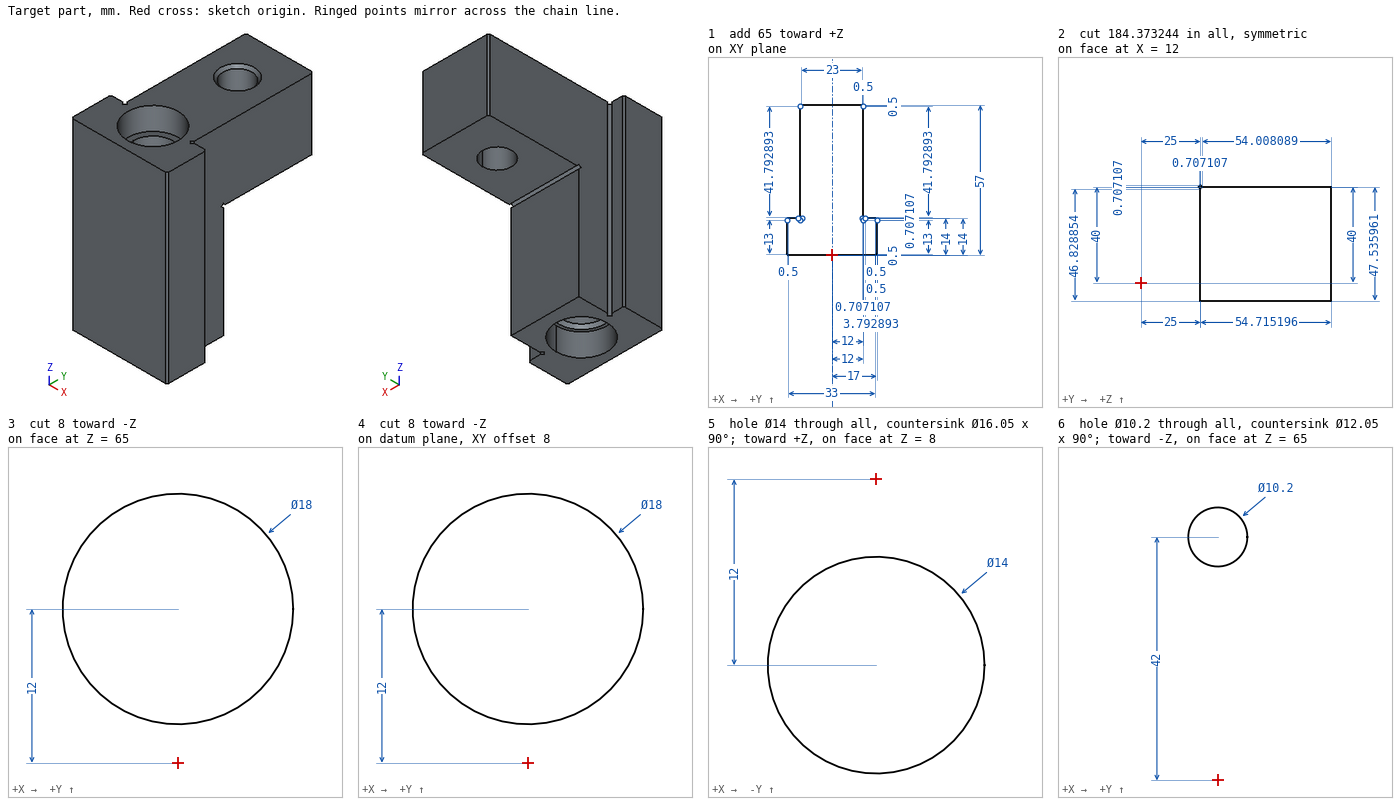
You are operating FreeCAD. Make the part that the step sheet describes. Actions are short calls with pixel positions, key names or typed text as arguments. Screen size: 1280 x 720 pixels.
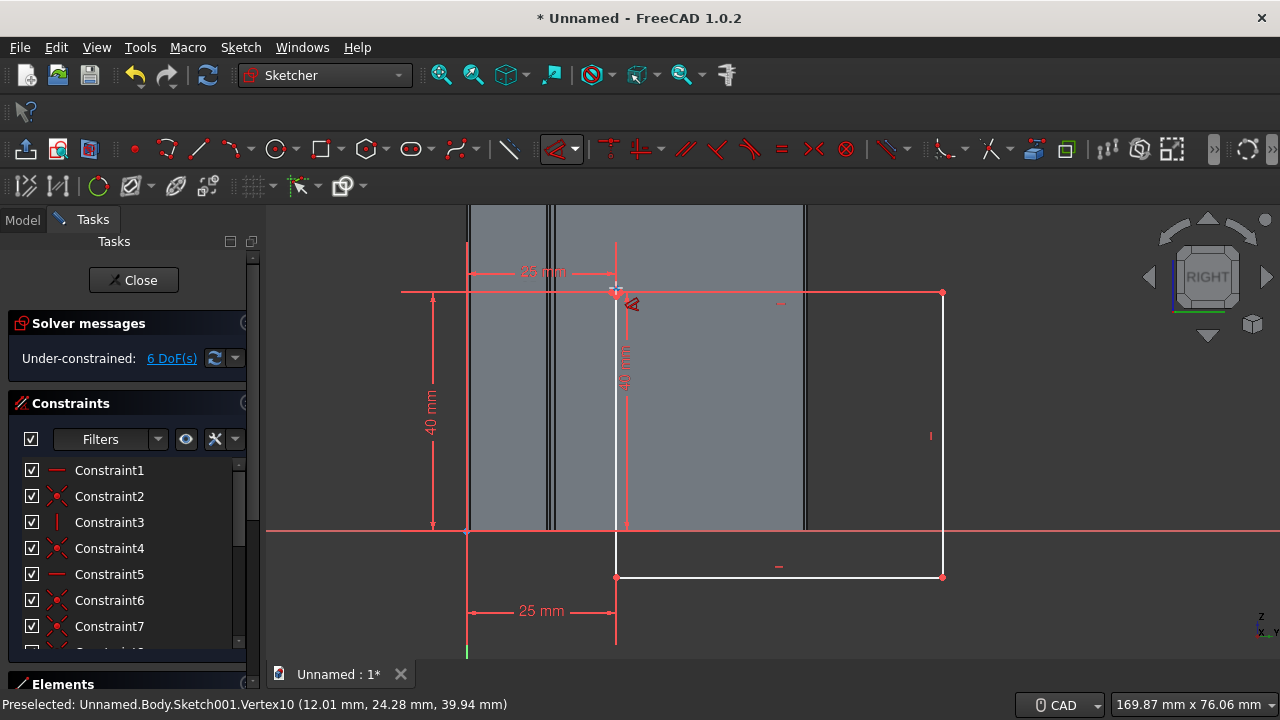
click(714, 578)
click(779, 612)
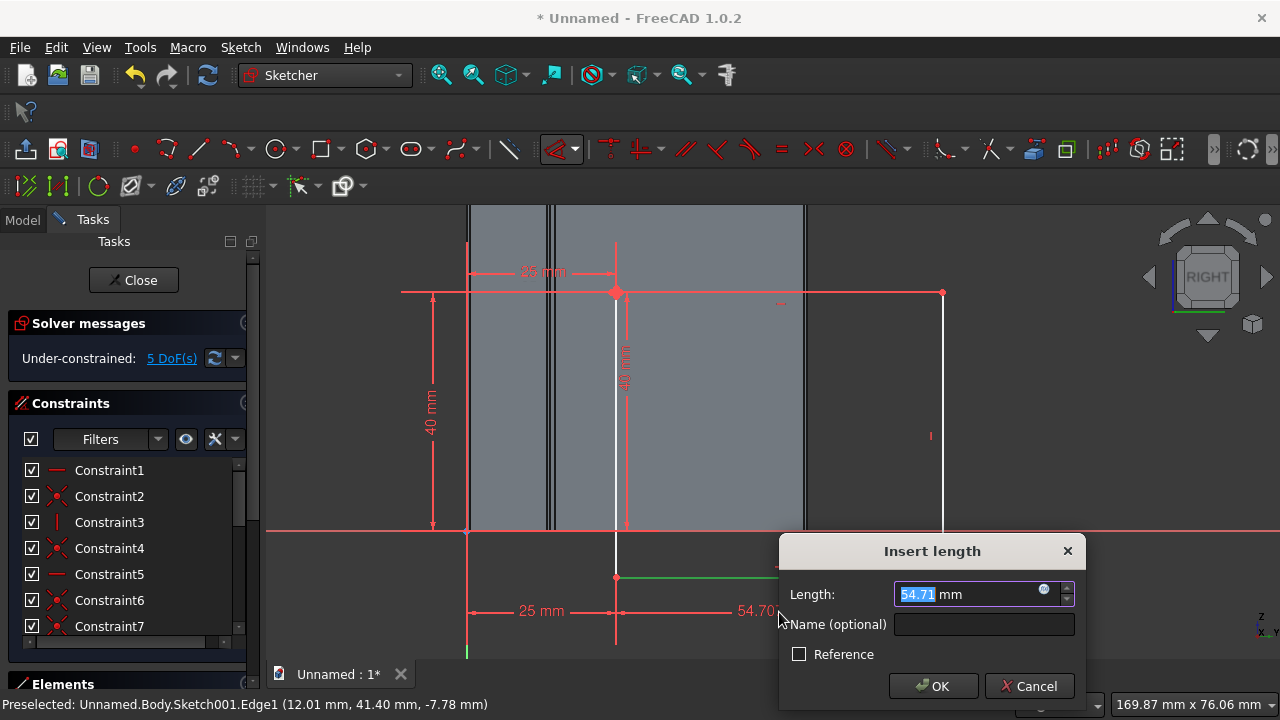
text(54.715196)
key(Return)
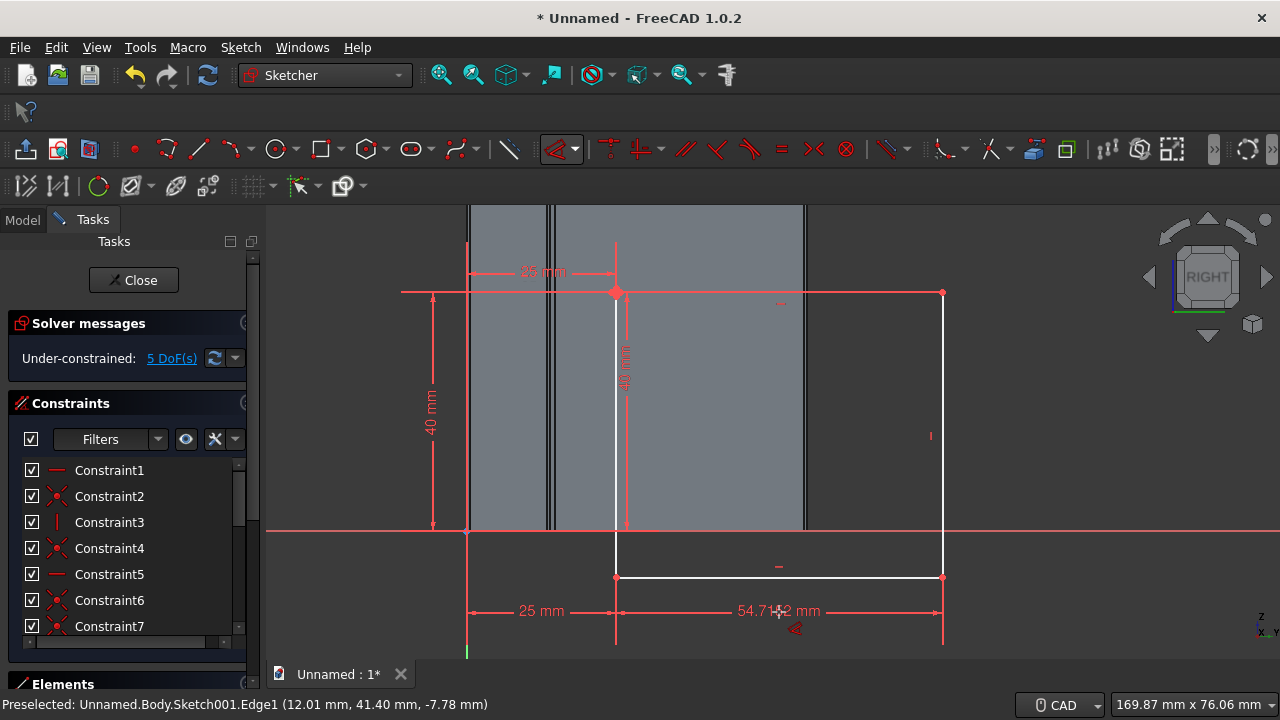
click(943, 492)
click(977, 435)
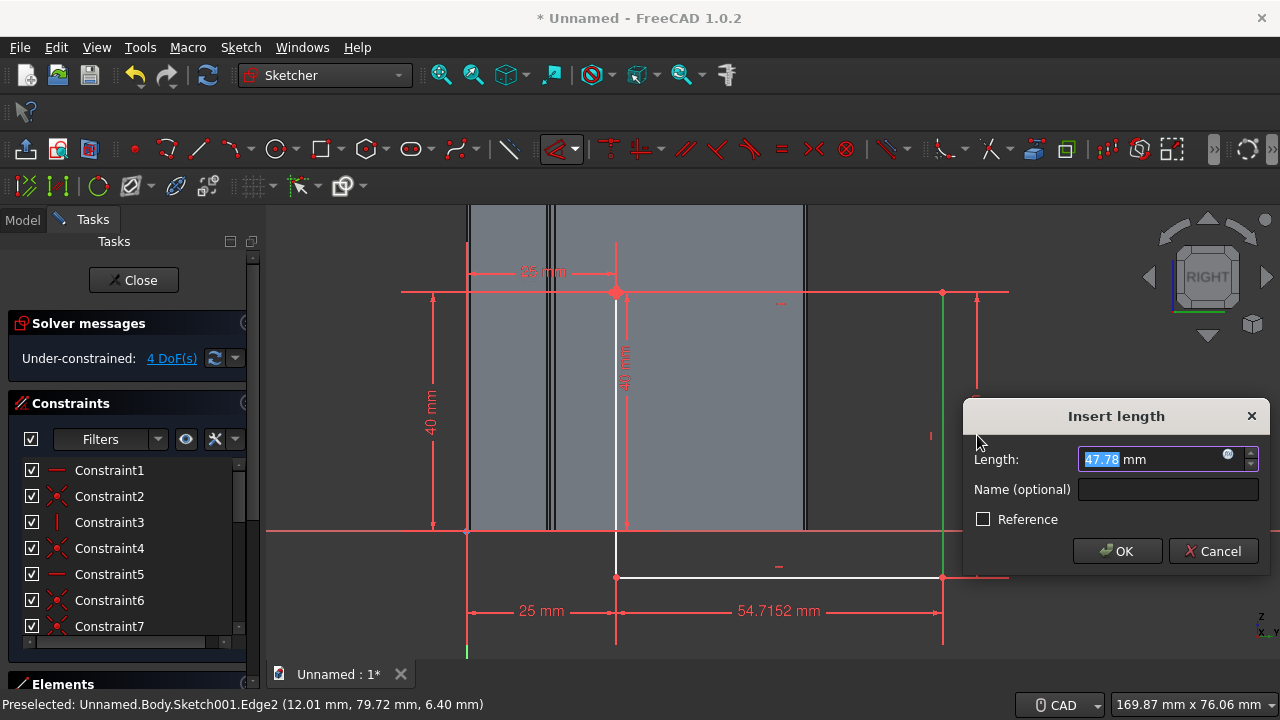
text(47.535961)
key(Return)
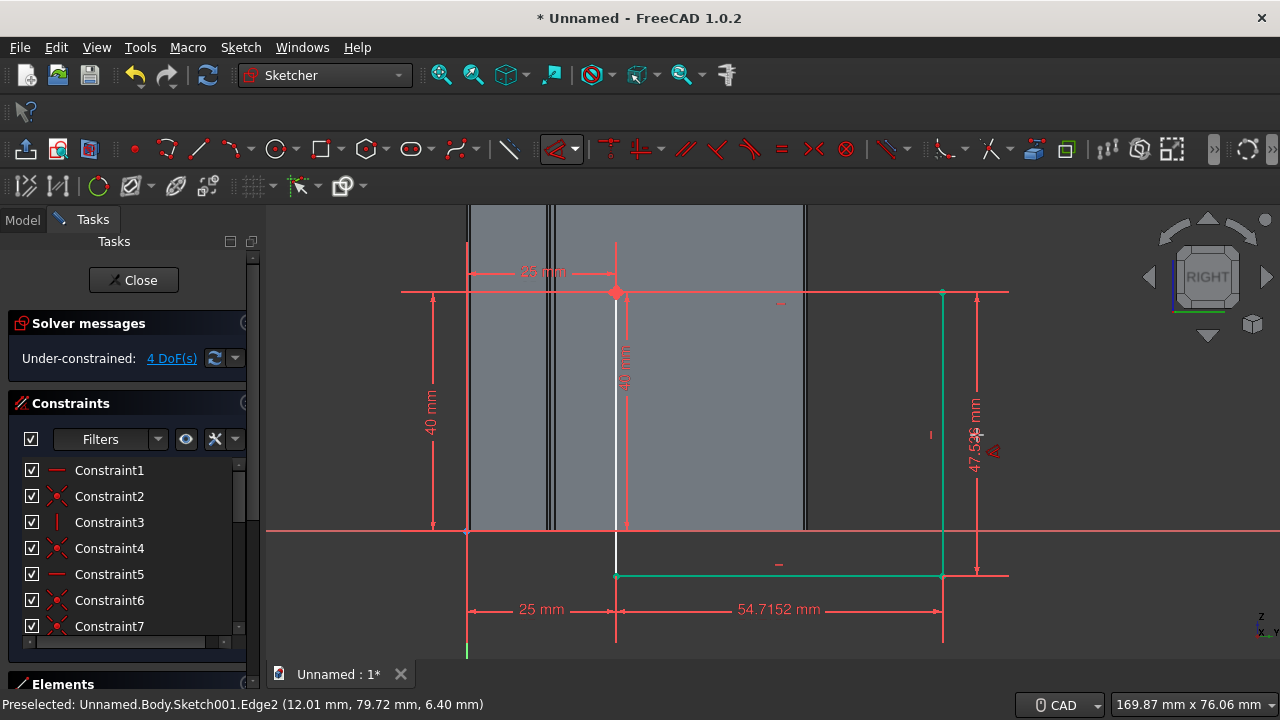
click(846, 292)
click(782, 258)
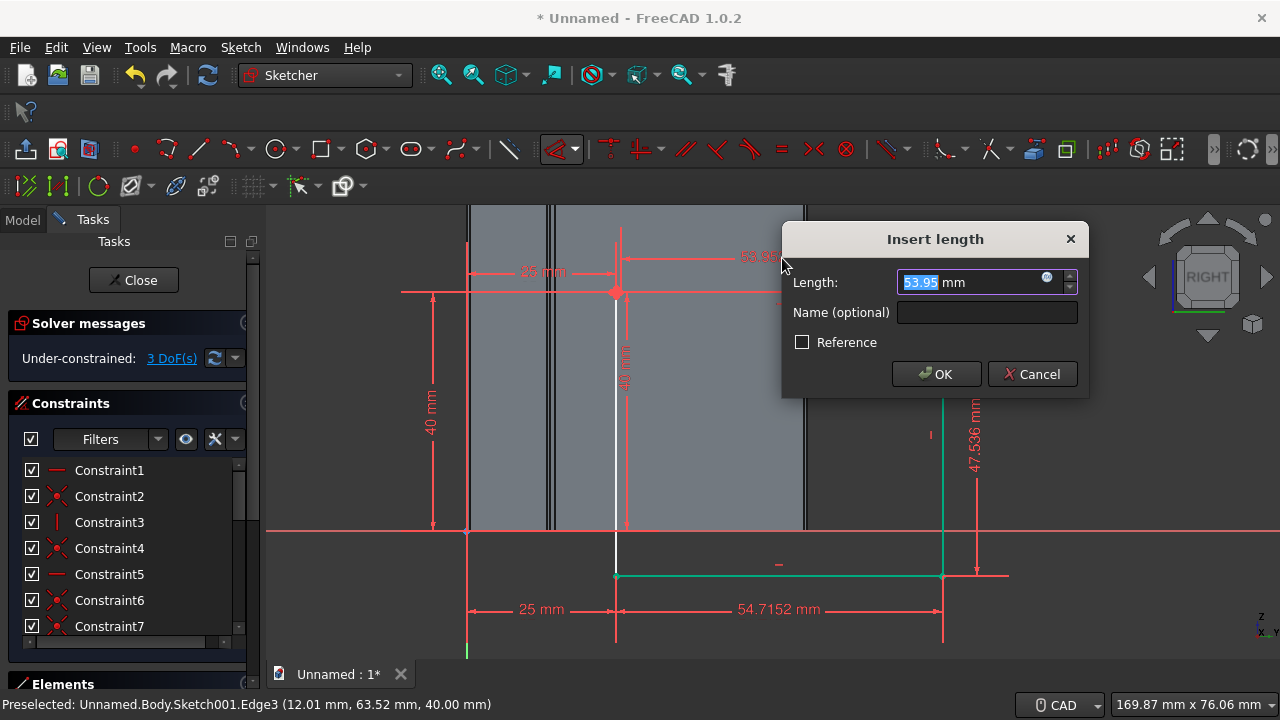
text(54.008089)
key(Return)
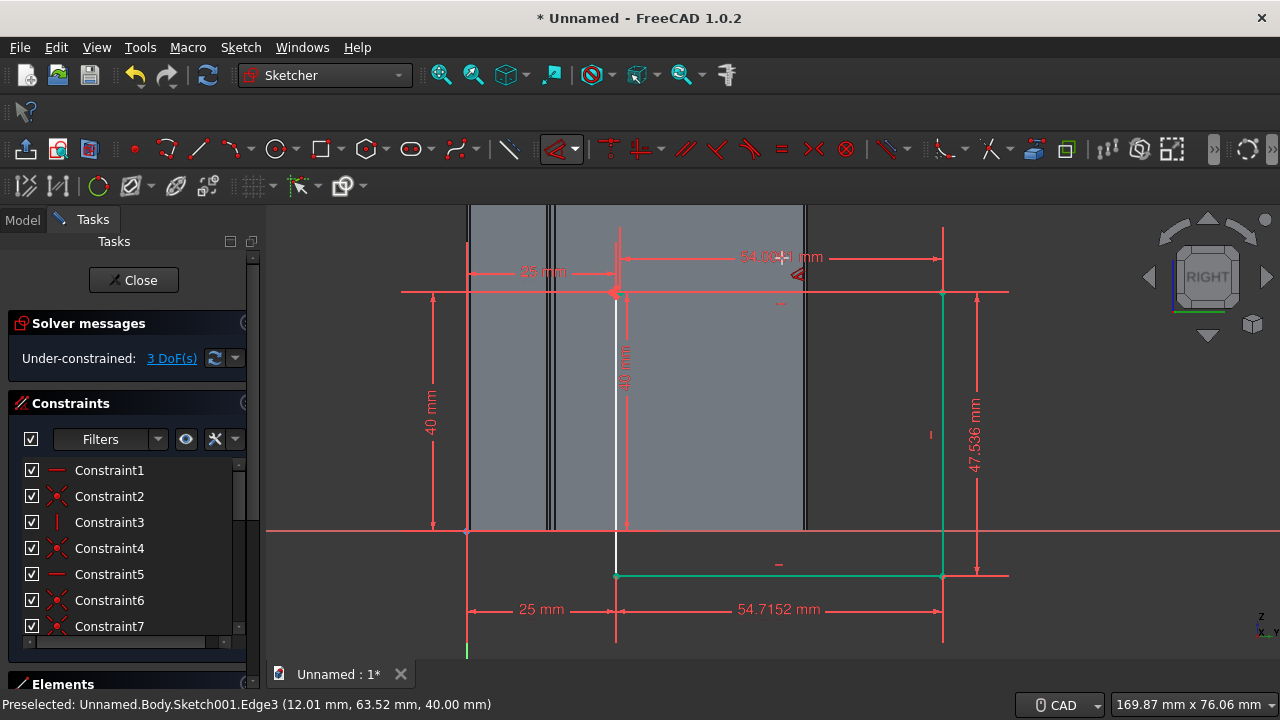
click(616, 381)
click(582, 437)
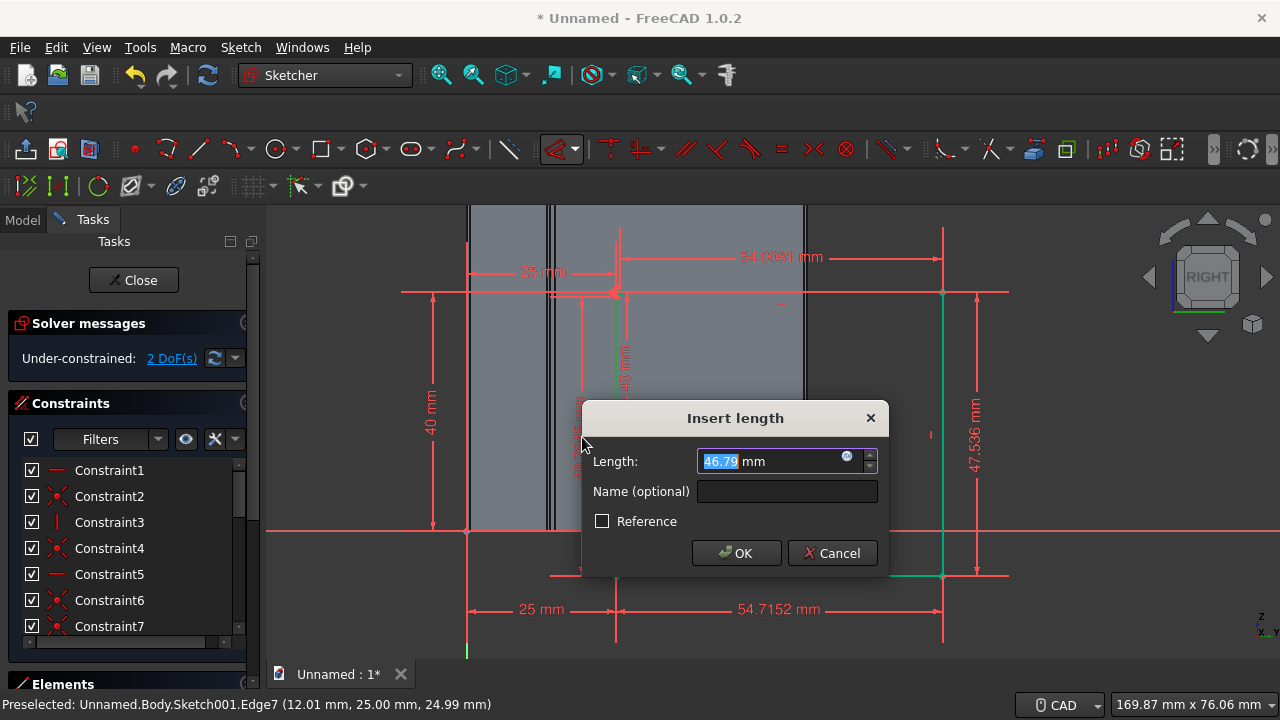
text(46.828854)
key(Return)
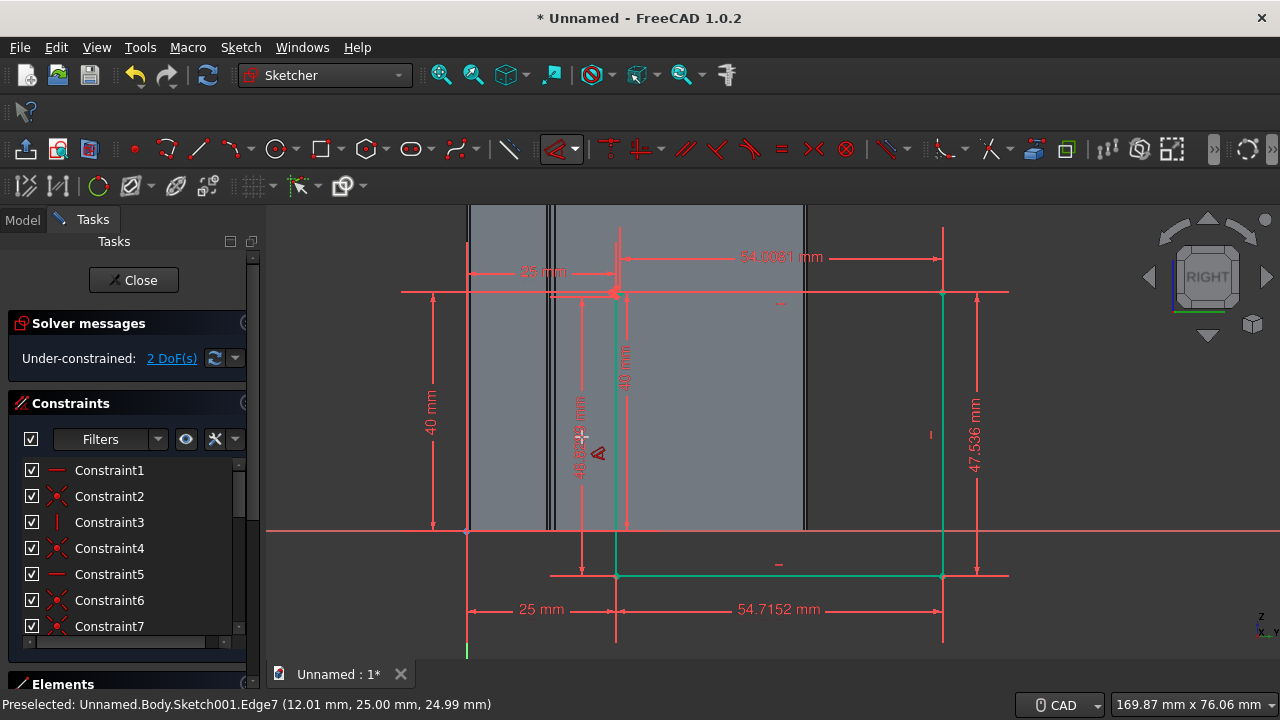
scroll(618, 290, up, 12)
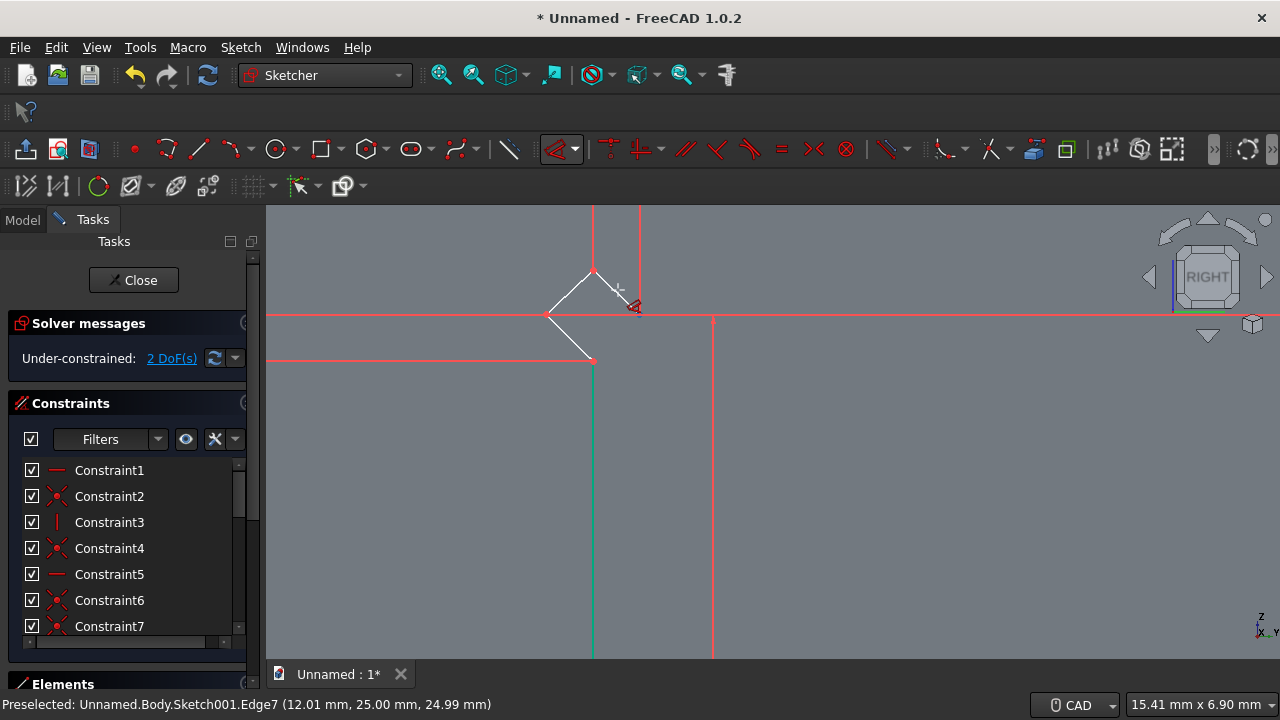
click(617, 293)
click(559, 282)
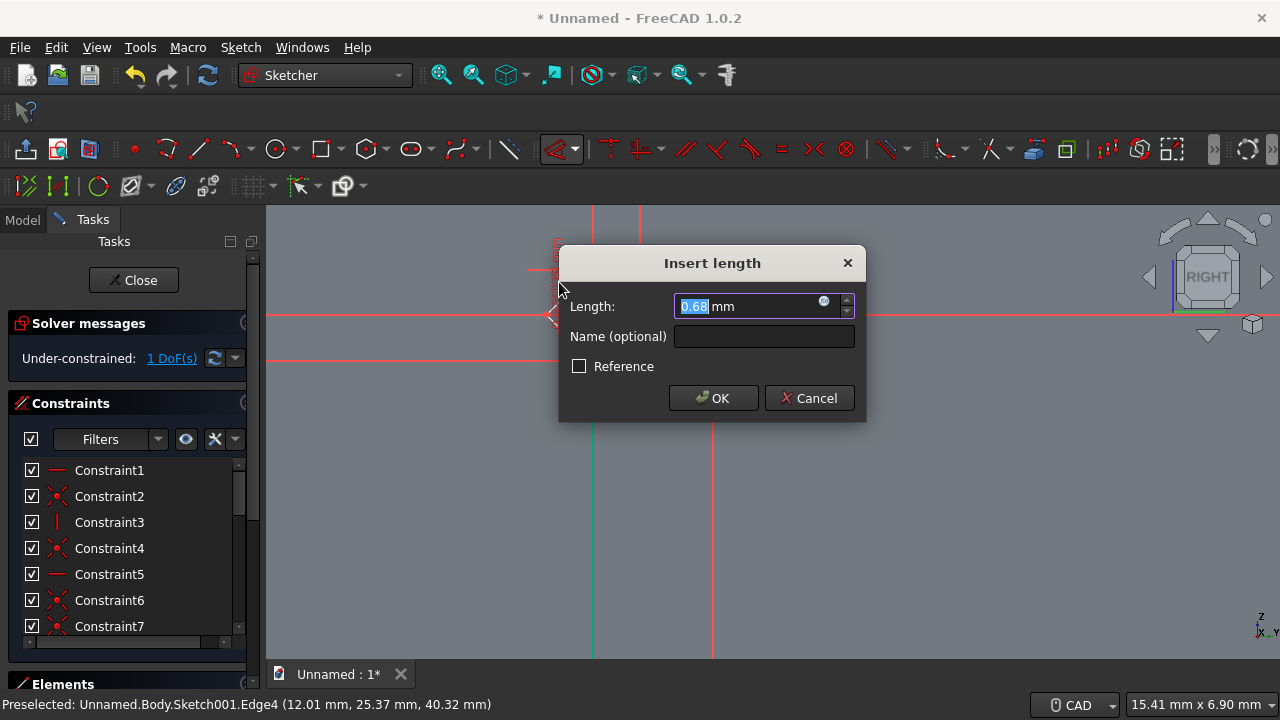
text(0.707107)
key(Return)